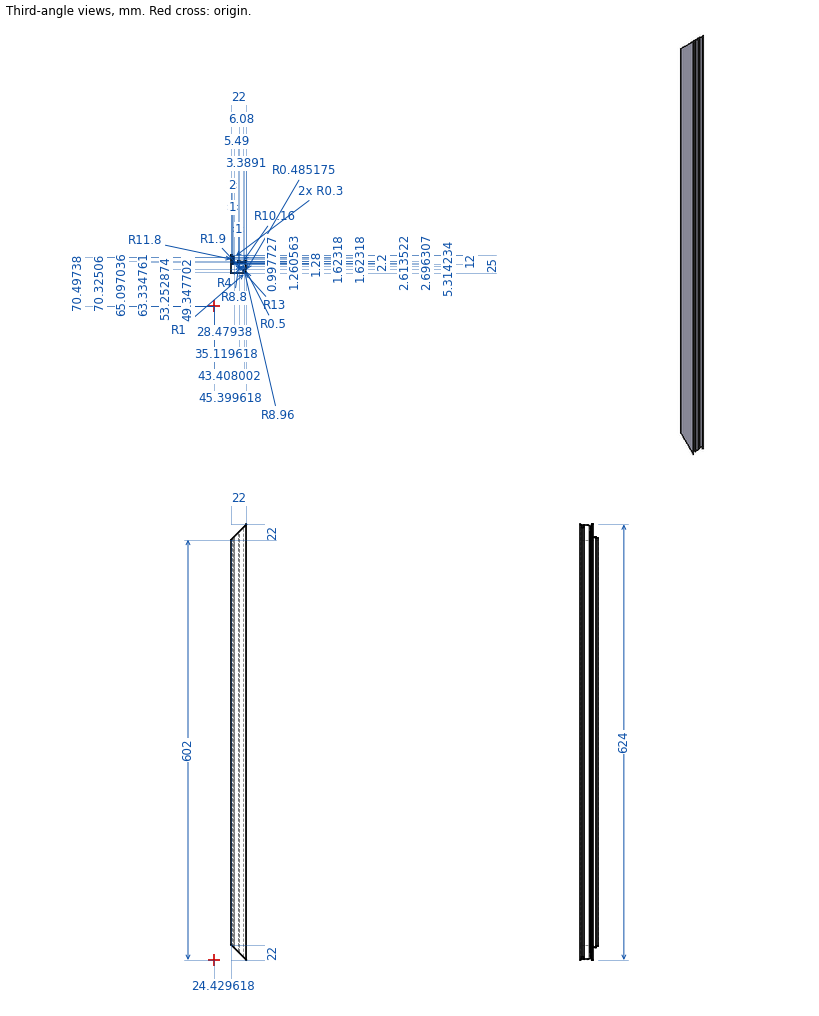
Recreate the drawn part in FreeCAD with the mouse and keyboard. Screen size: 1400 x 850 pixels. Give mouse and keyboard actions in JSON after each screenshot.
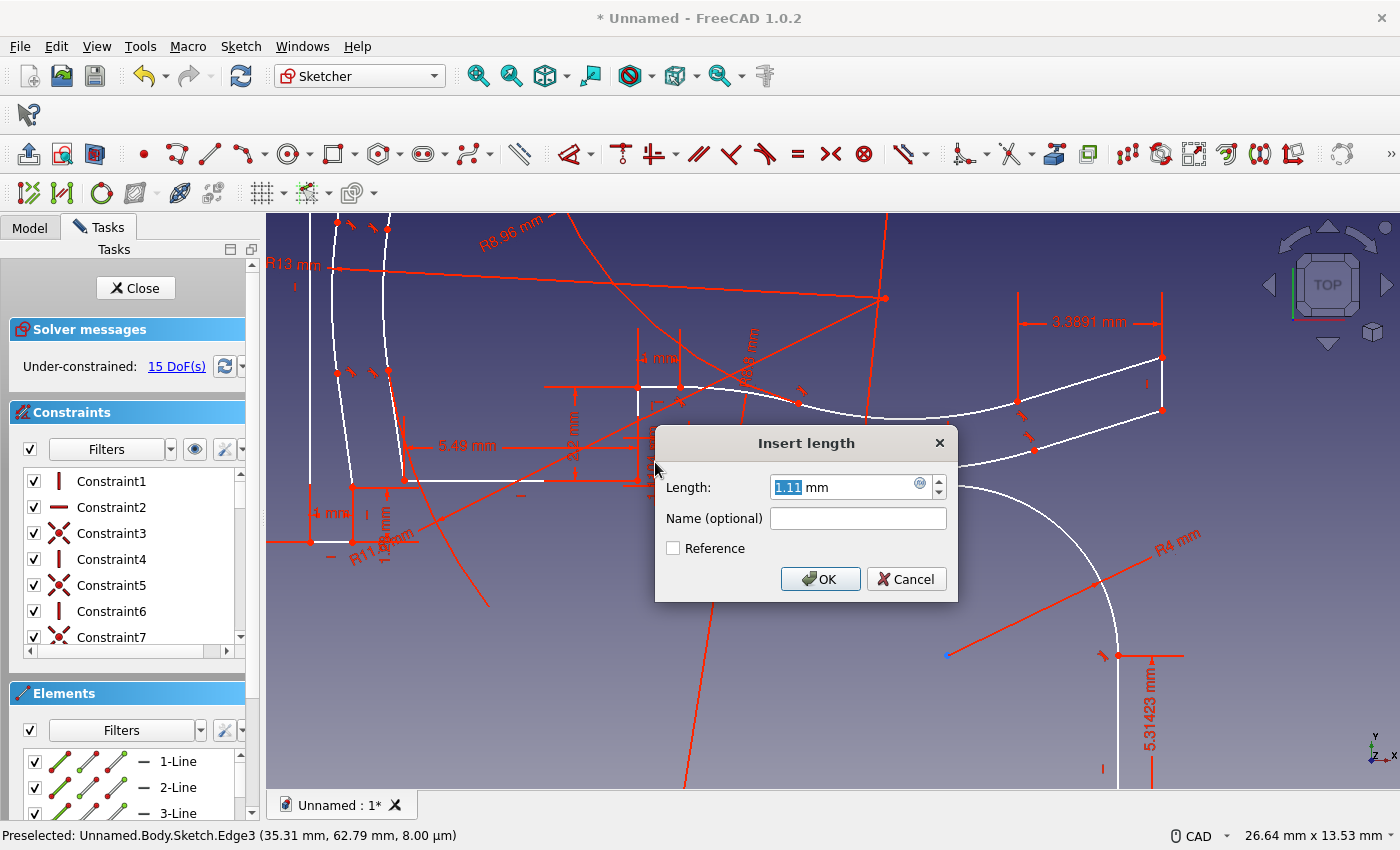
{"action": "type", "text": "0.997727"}
{"action": "key", "text": "Return"}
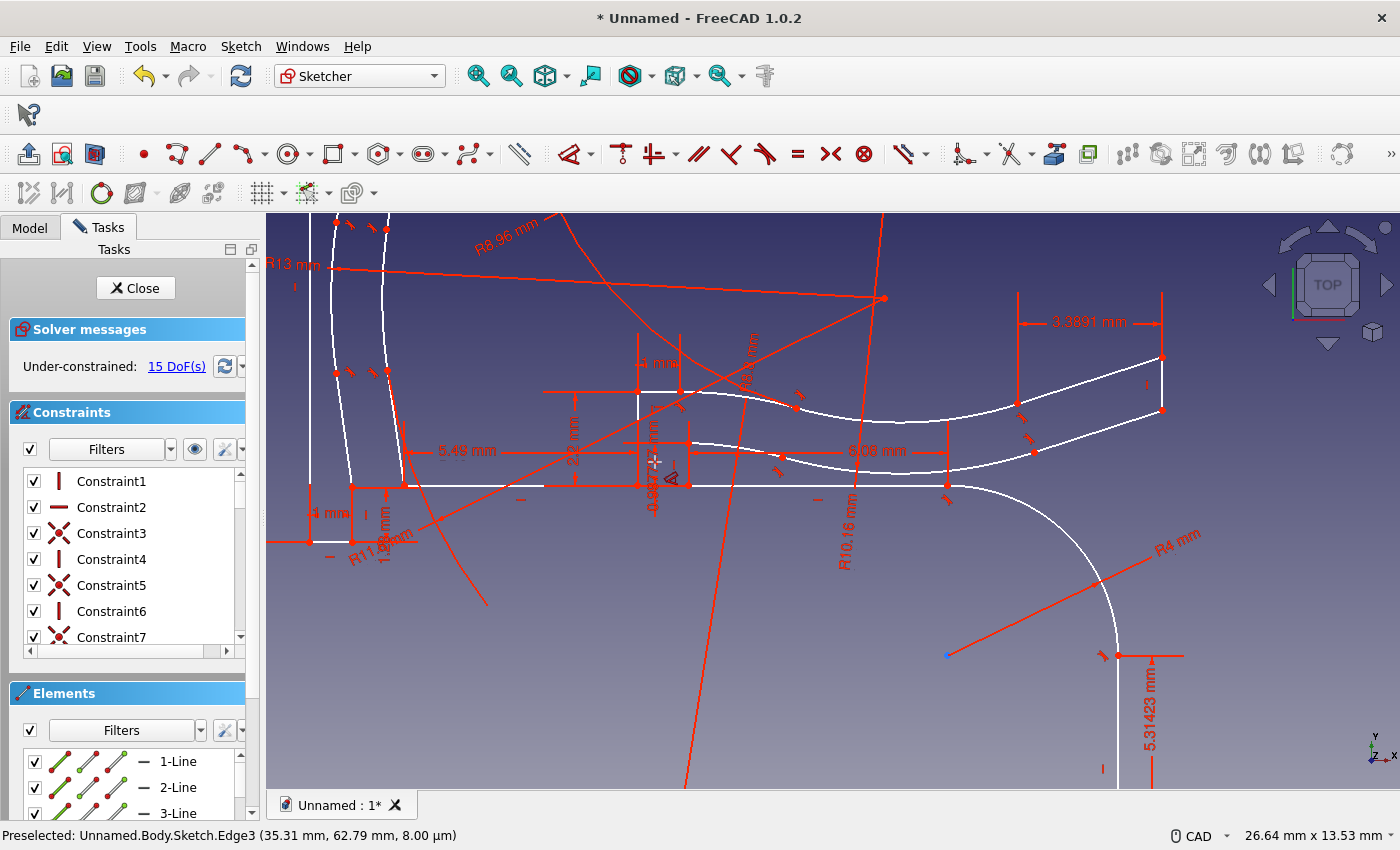
{"action": "left_click", "coordinate": [1162, 395]}
{"action": "left_click", "coordinate": [1196, 384]}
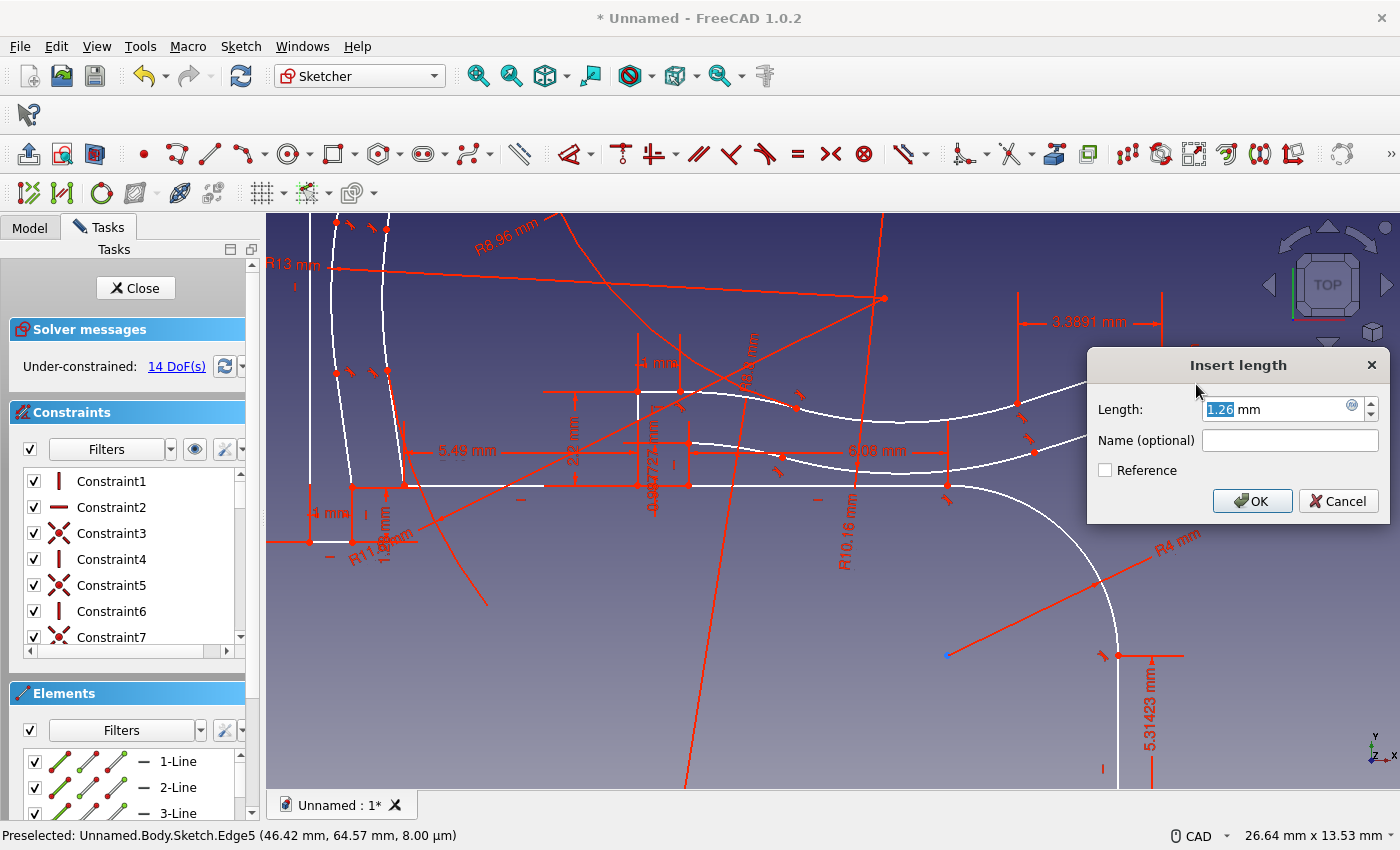
{"action": "type", "text": "1.260563"}
{"action": "key", "text": "Return"}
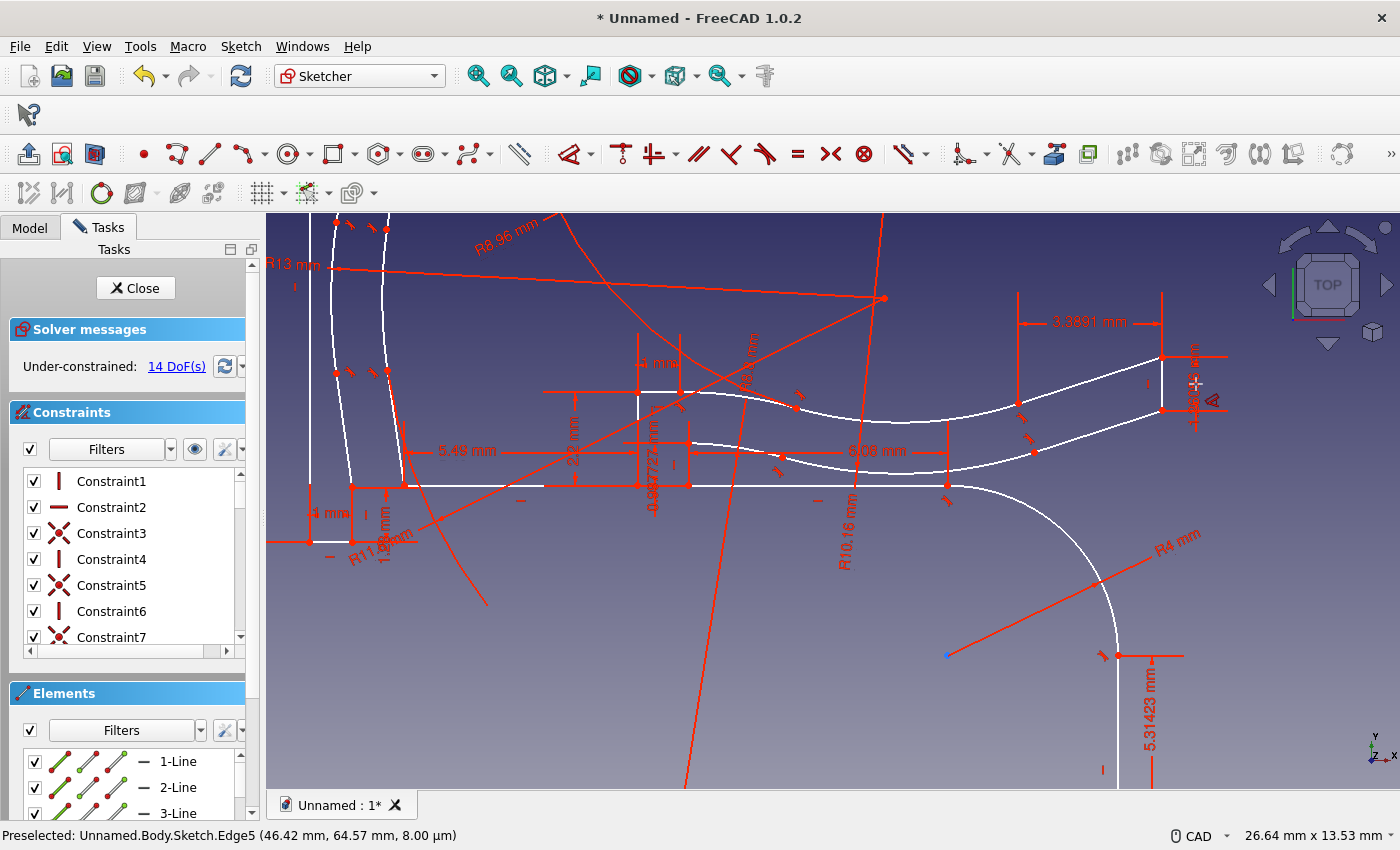
{"action": "scroll", "coordinate": [805, 466], "scroll_direction": "down", "scroll_amount": 5}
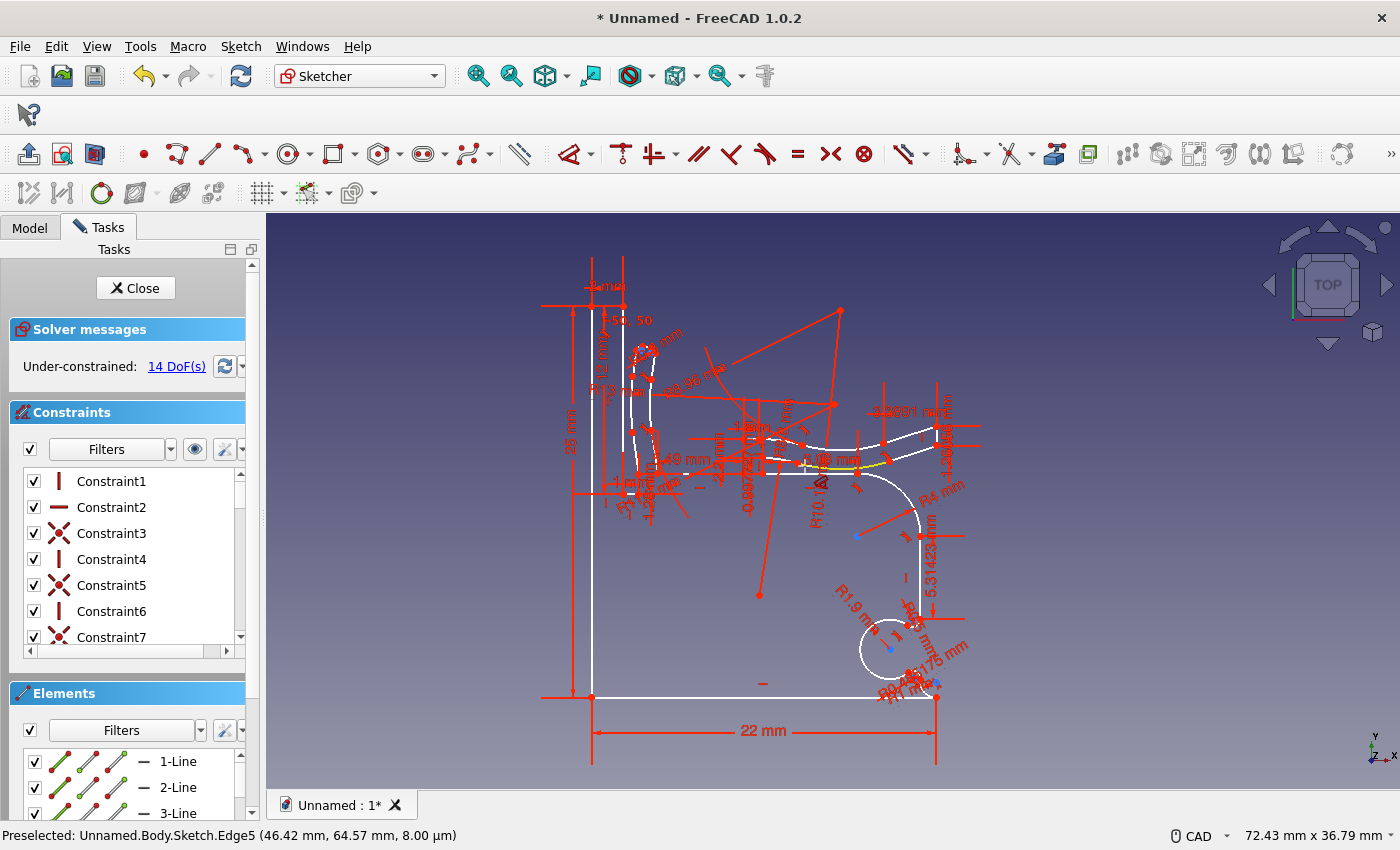
{"action": "scroll", "coordinate": [653, 372], "scroll_direction": "up", "scroll_amount": 3}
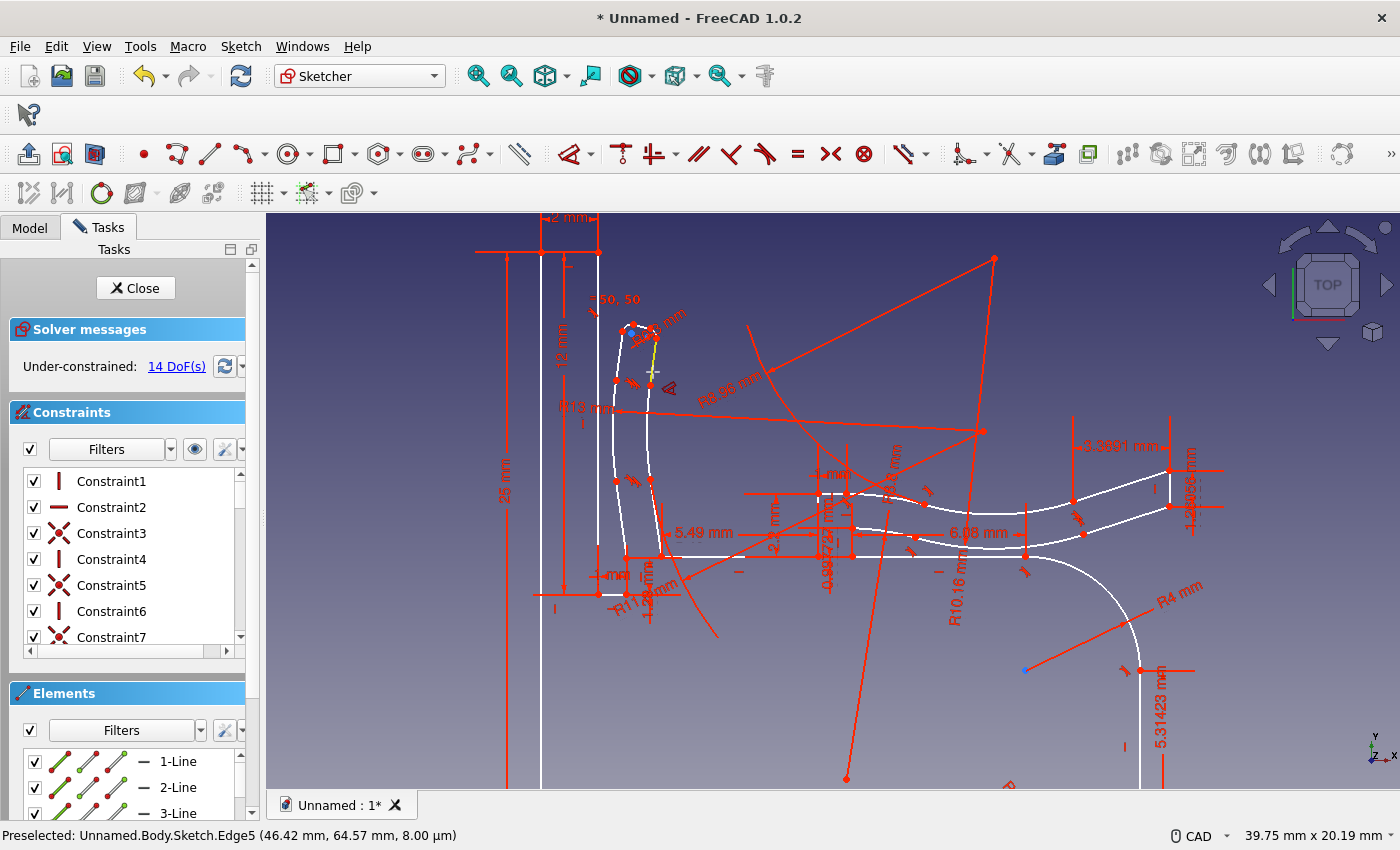
{"action": "left_click", "coordinate": [652, 371]}
{"action": "left_click", "coordinate": [690, 362]}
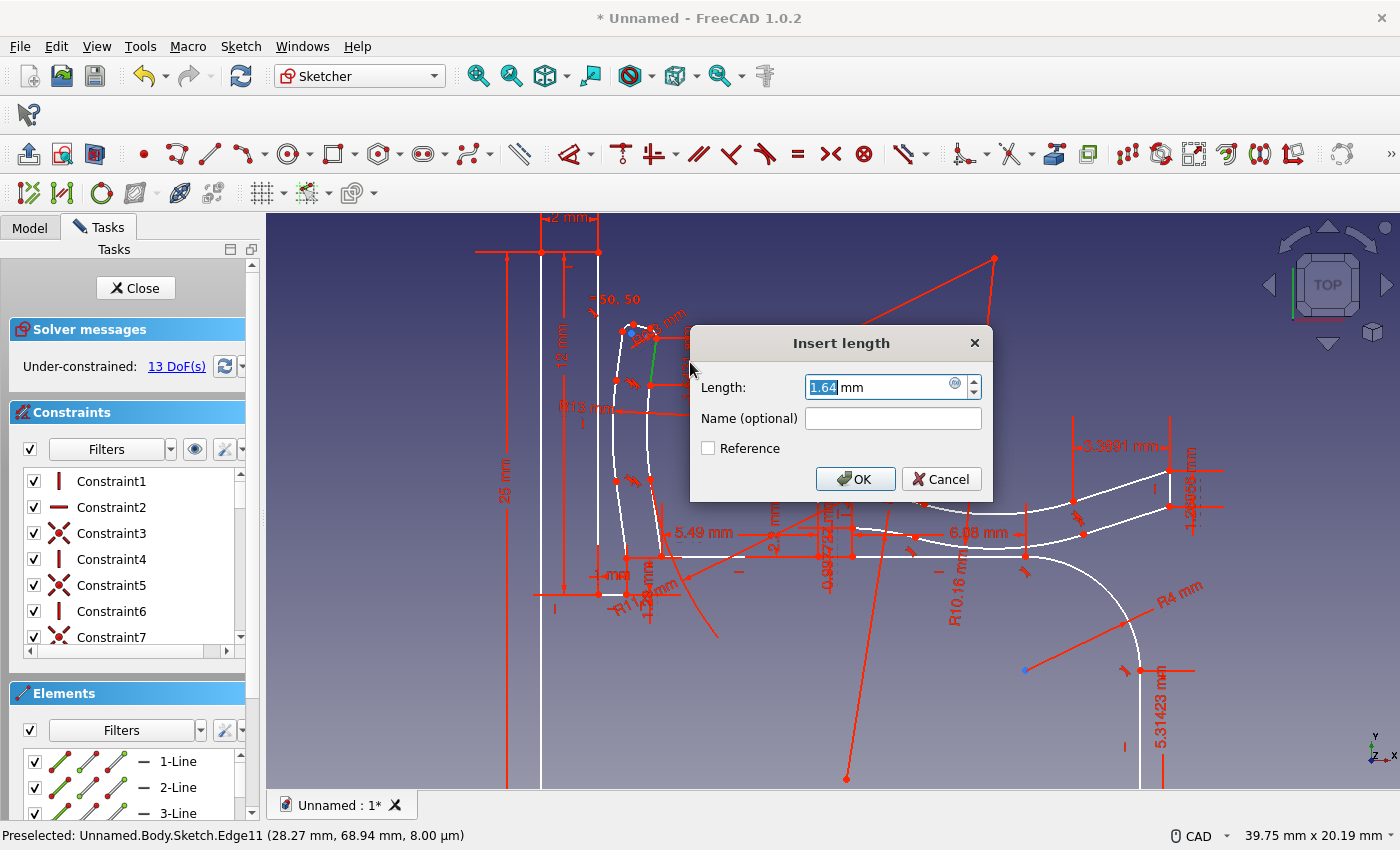
{"action": "type", "text": "1.62318"}
{"action": "key", "text": "Return"}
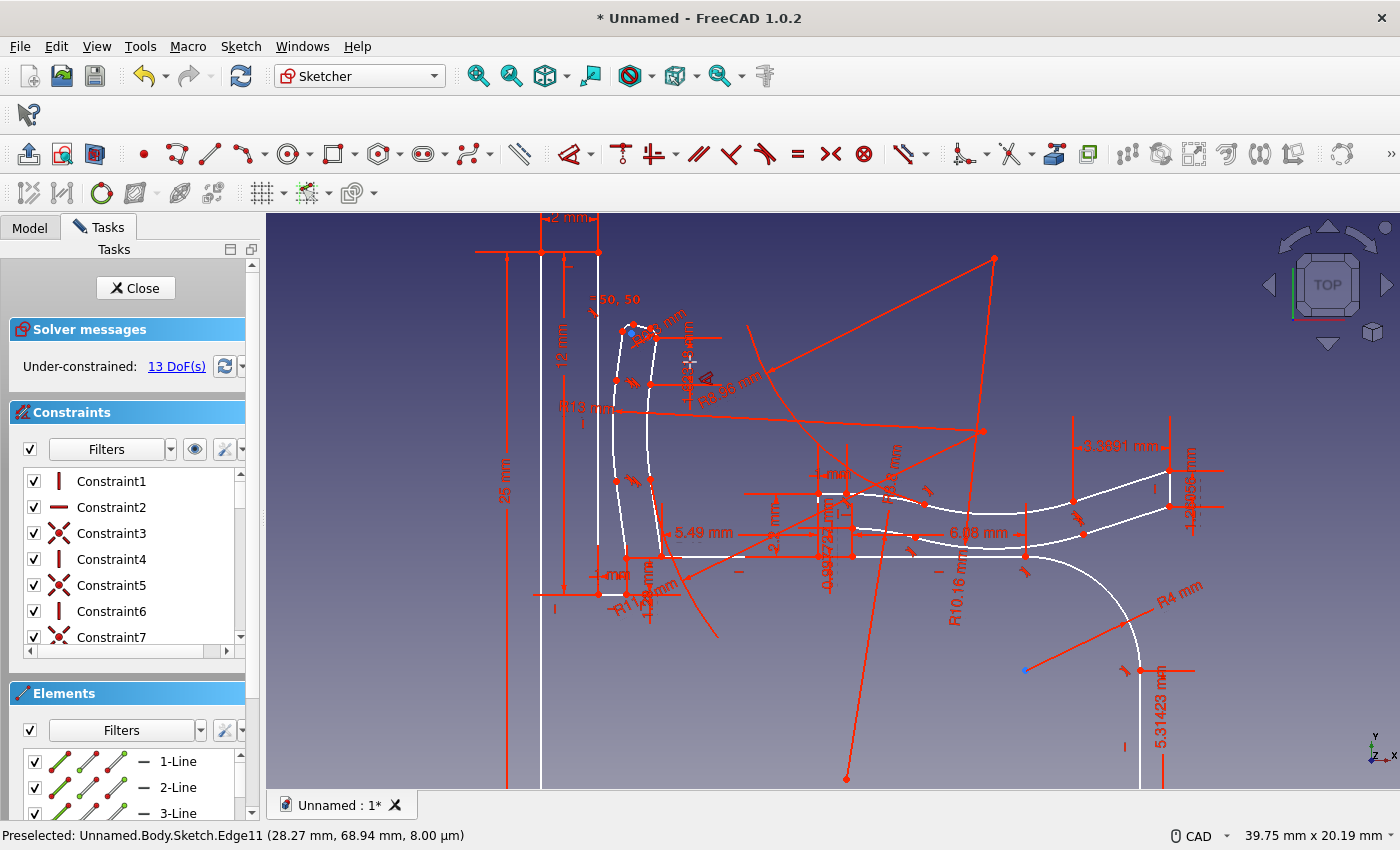
{"action": "left_click", "coordinate": [621, 346]}
{"action": "left_click", "coordinate": [582, 367]}